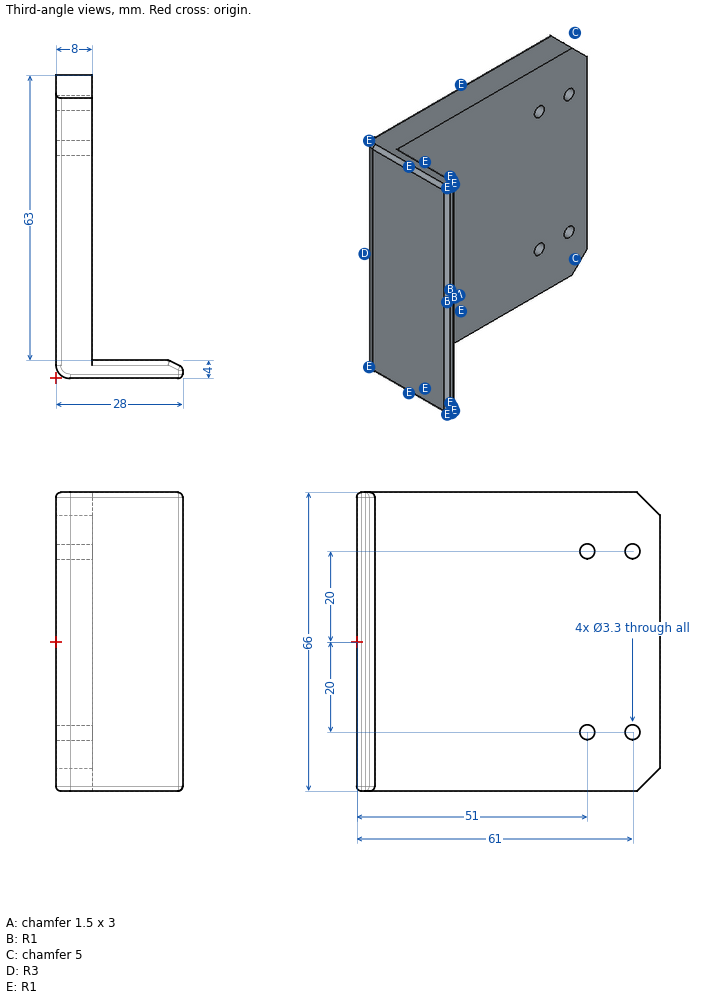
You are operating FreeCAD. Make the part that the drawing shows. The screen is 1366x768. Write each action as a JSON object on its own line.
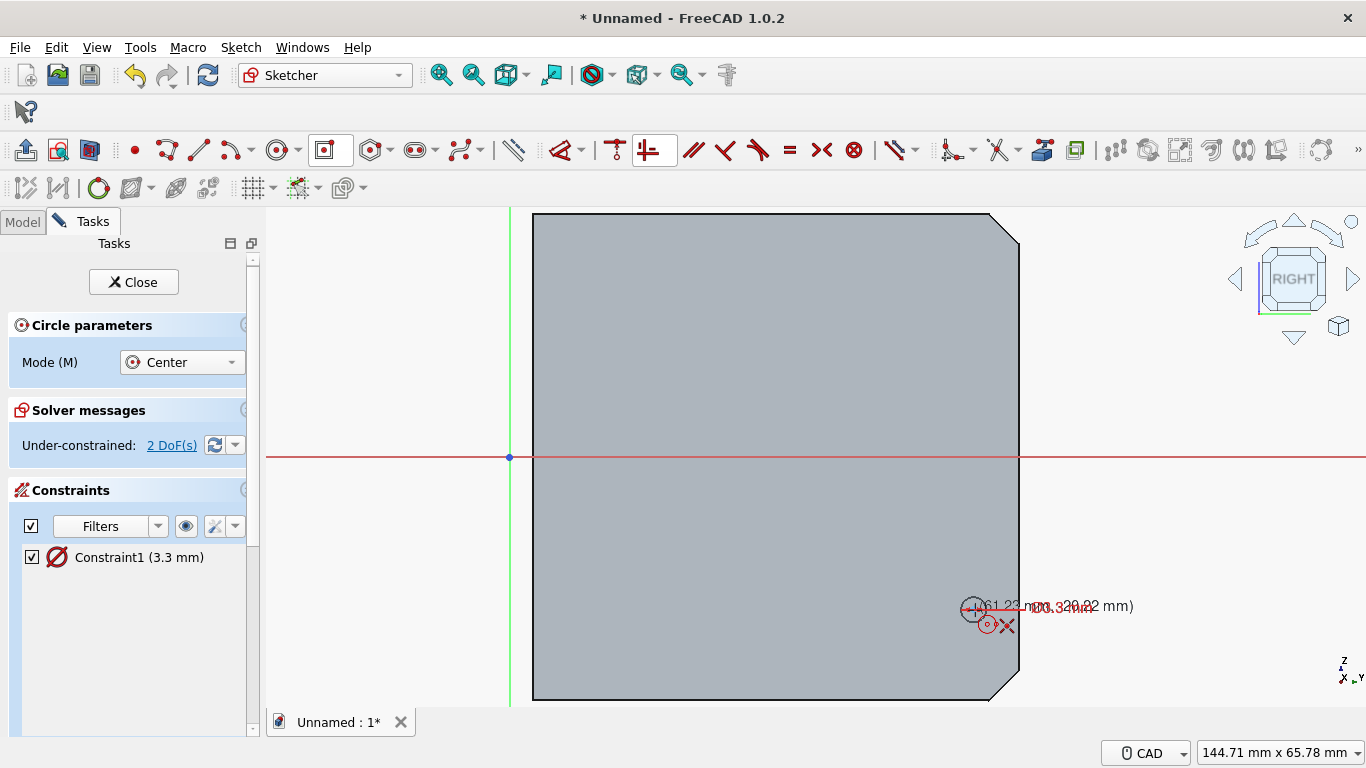
{"action": "scroll", "coordinate": [974, 305], "scroll_direction": "up", "scroll_amount": 3}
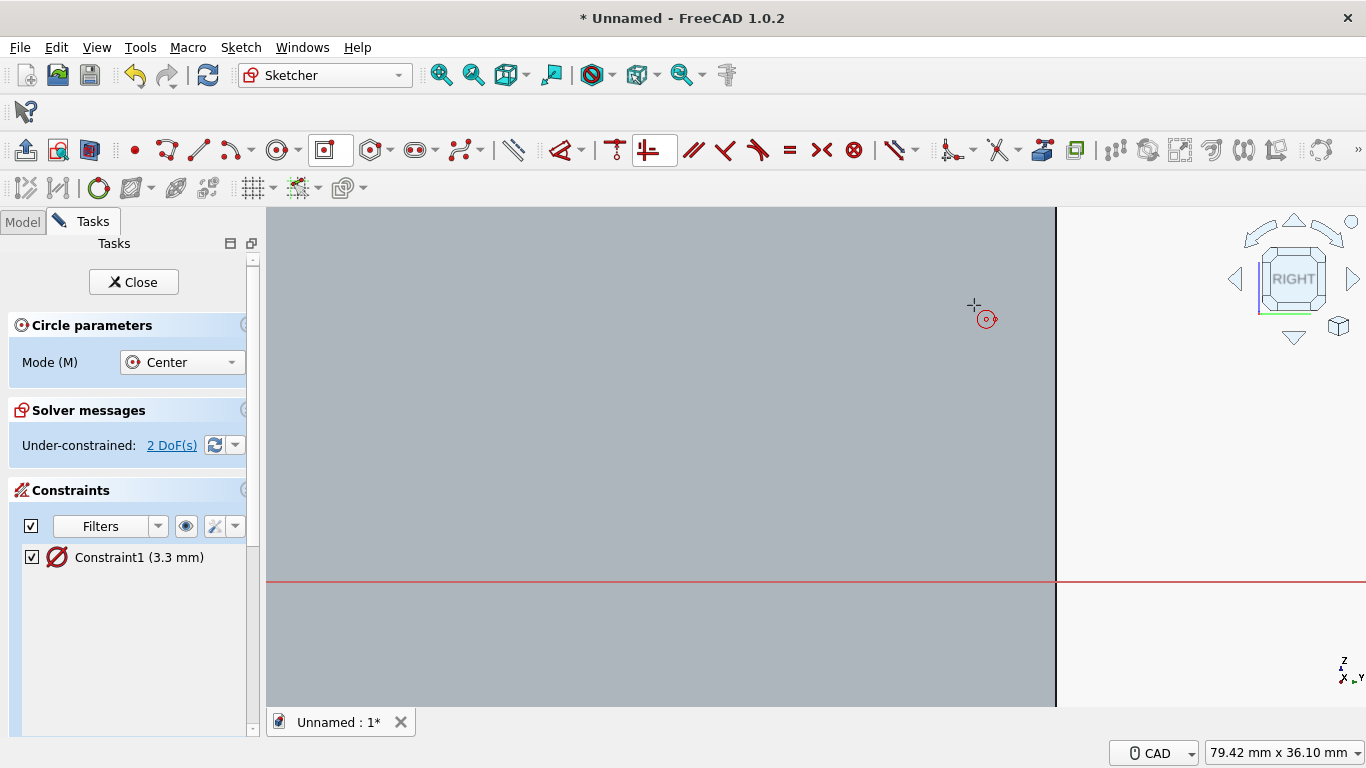
{"action": "left_click", "coordinate": [973, 305]}
{"action": "mouse_move", "coordinate": [989, 289]}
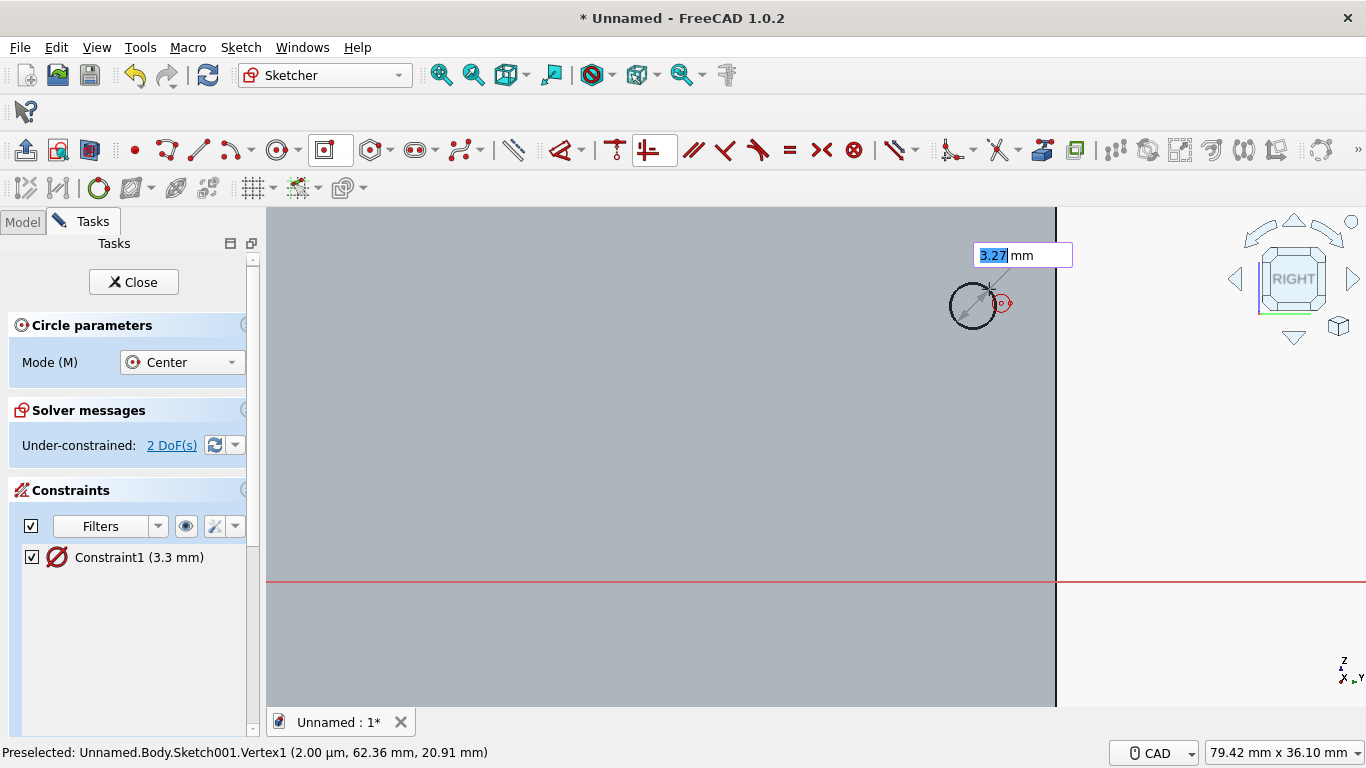
{"action": "type", "text": "3.3"}
{"action": "key", "text": "Return"}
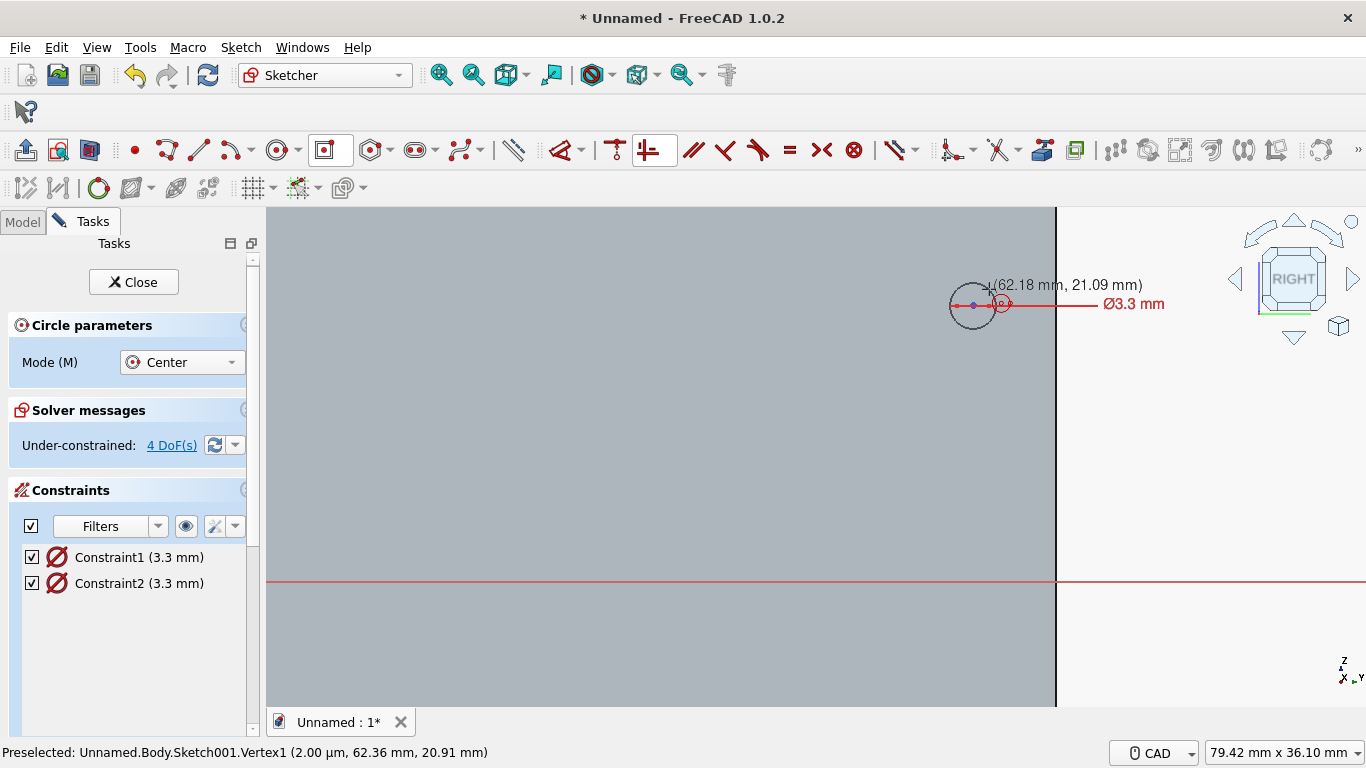
{"action": "scroll", "coordinate": [974, 305], "scroll_direction": "down", "scroll_amount": 3}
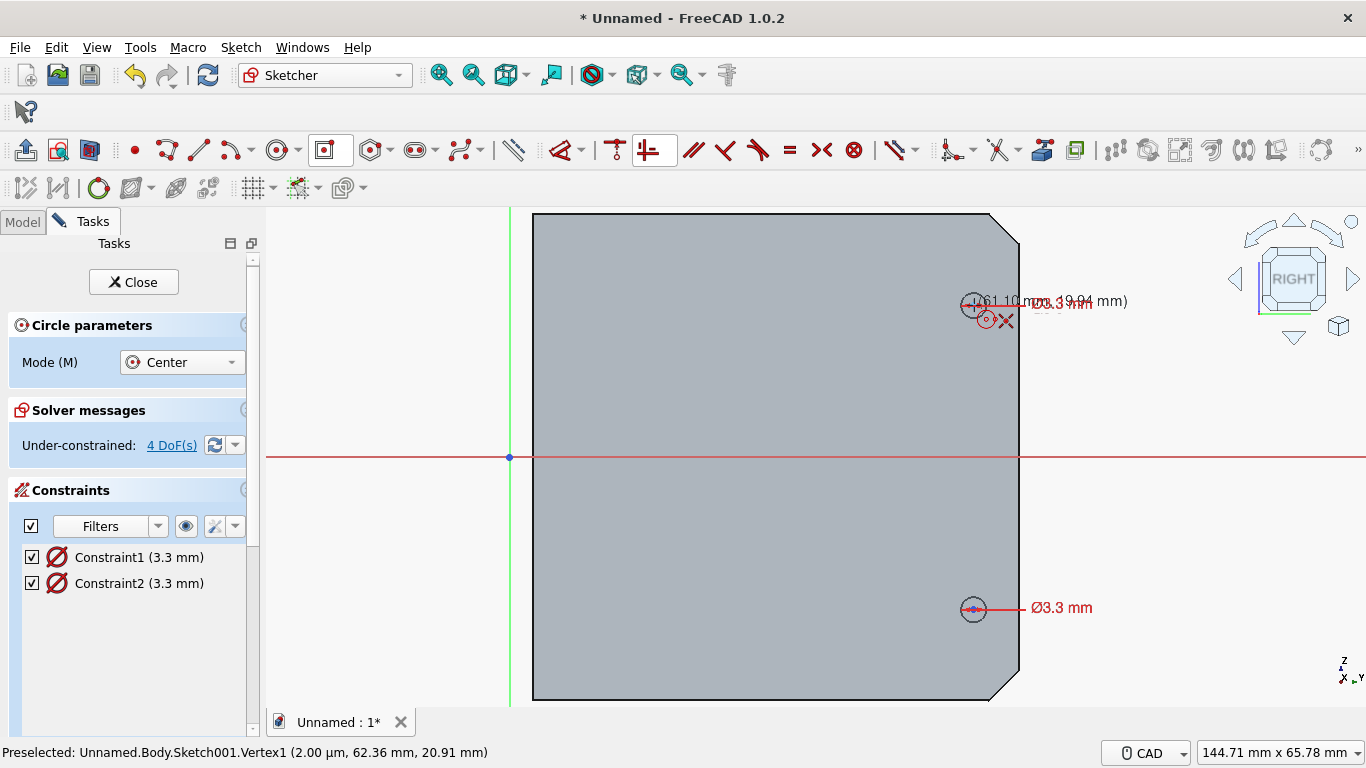
{"action": "scroll", "coordinate": [898, 609], "scroll_direction": "up", "scroll_amount": 3}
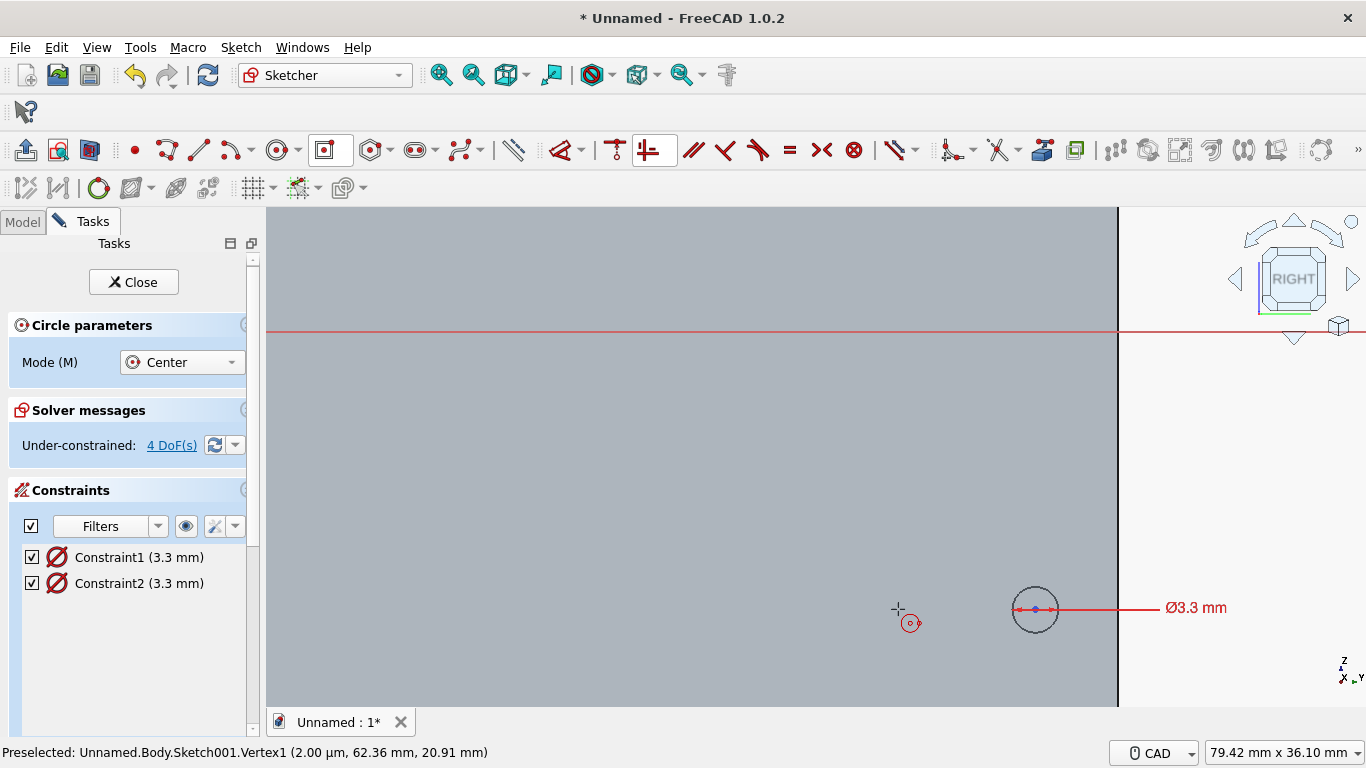
{"action": "left_click", "coordinate": [897, 609]}
{"action": "mouse_move", "coordinate": [913, 593]}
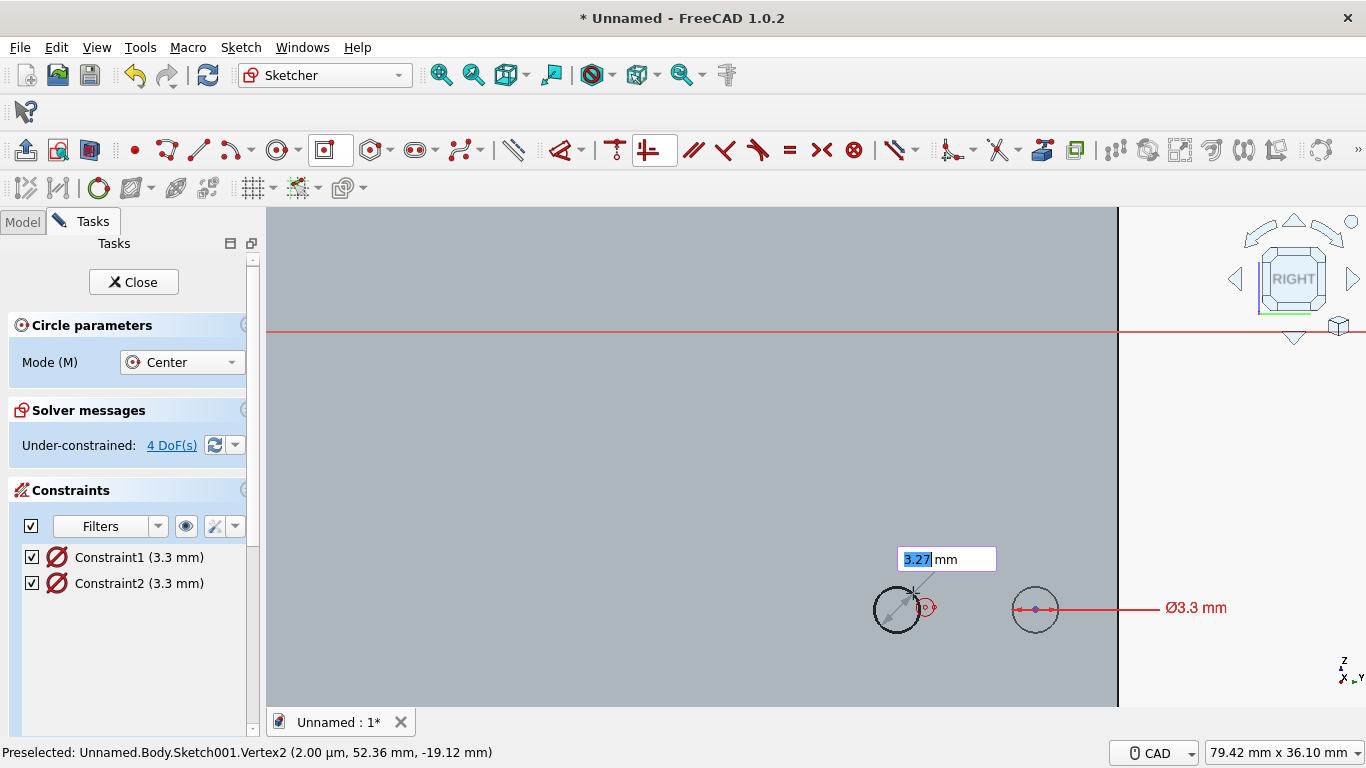
{"action": "type", "text": "3.3"}
{"action": "key", "text": "Return"}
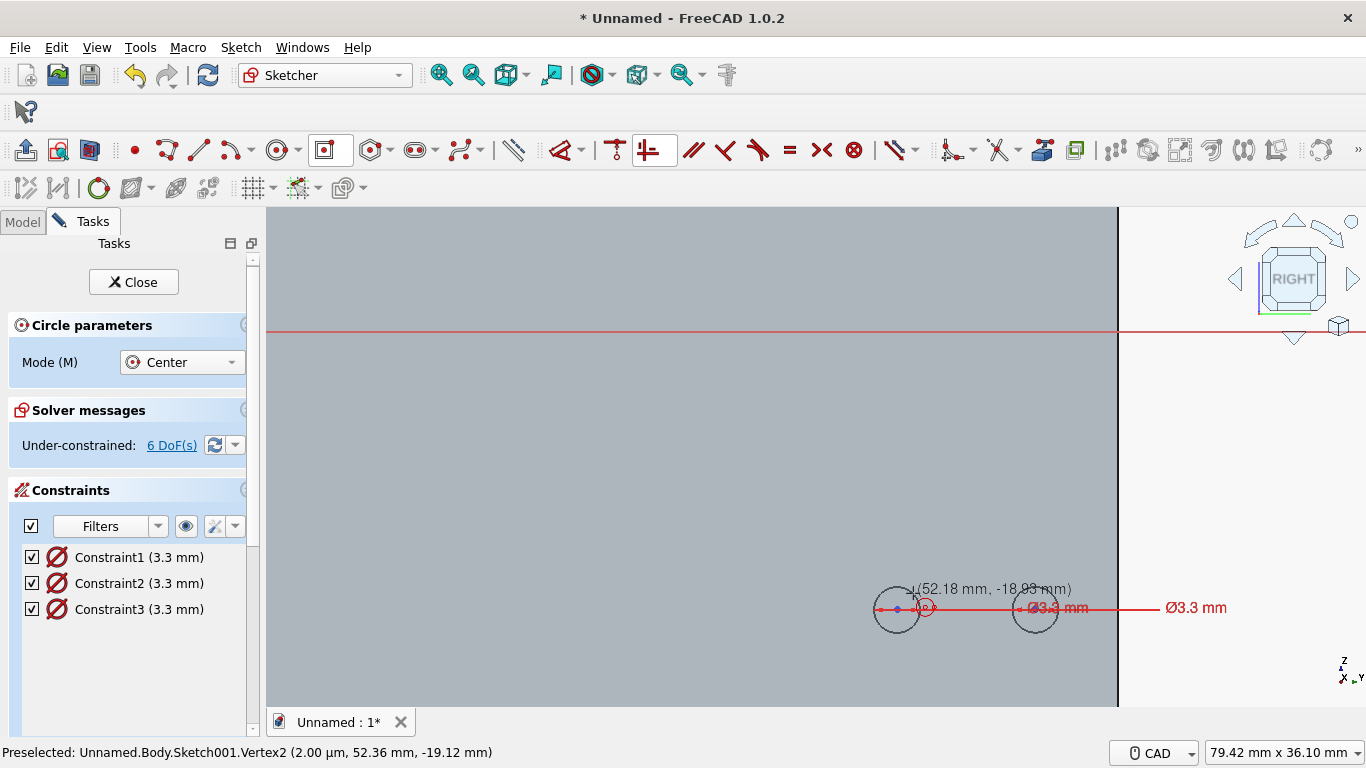
{"action": "scroll", "coordinate": [898, 609], "scroll_direction": "down", "scroll_amount": 3}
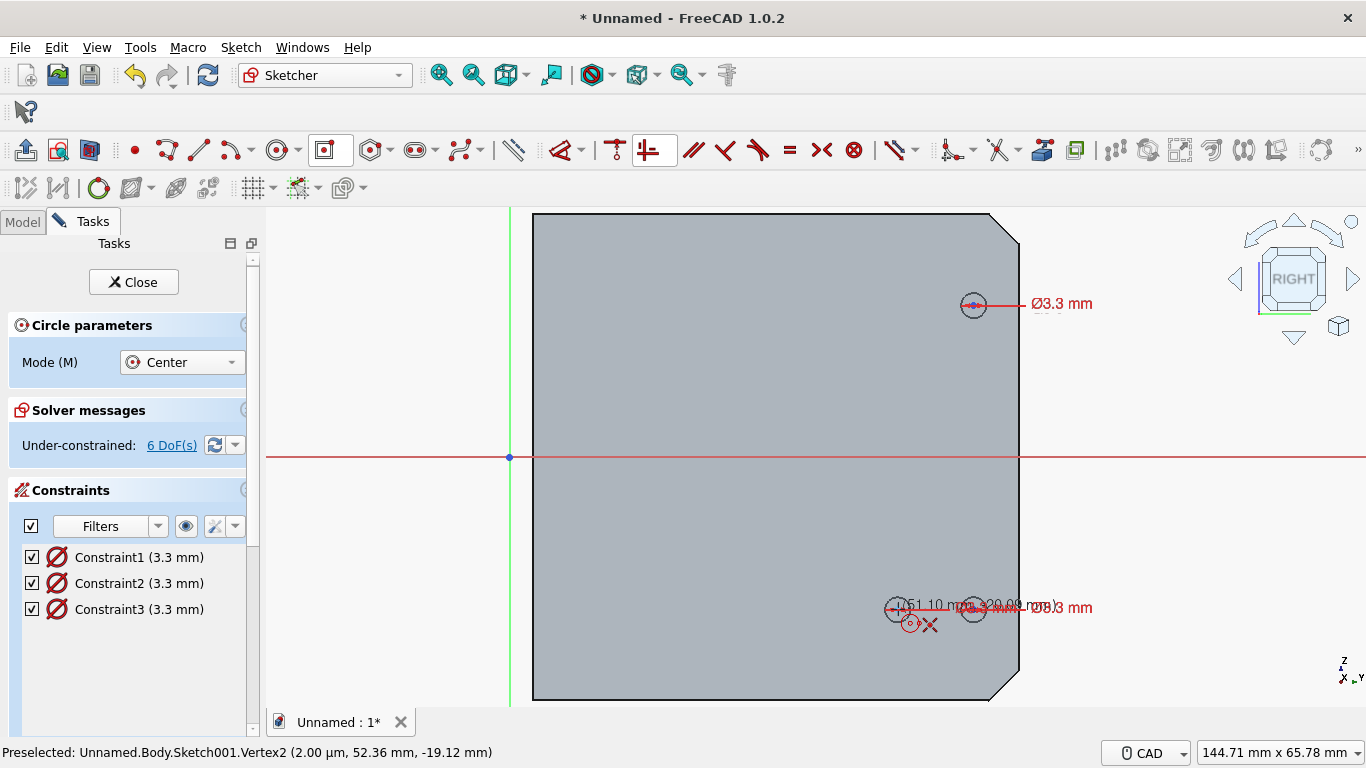
{"action": "scroll", "coordinate": [898, 305], "scroll_direction": "up", "scroll_amount": 3}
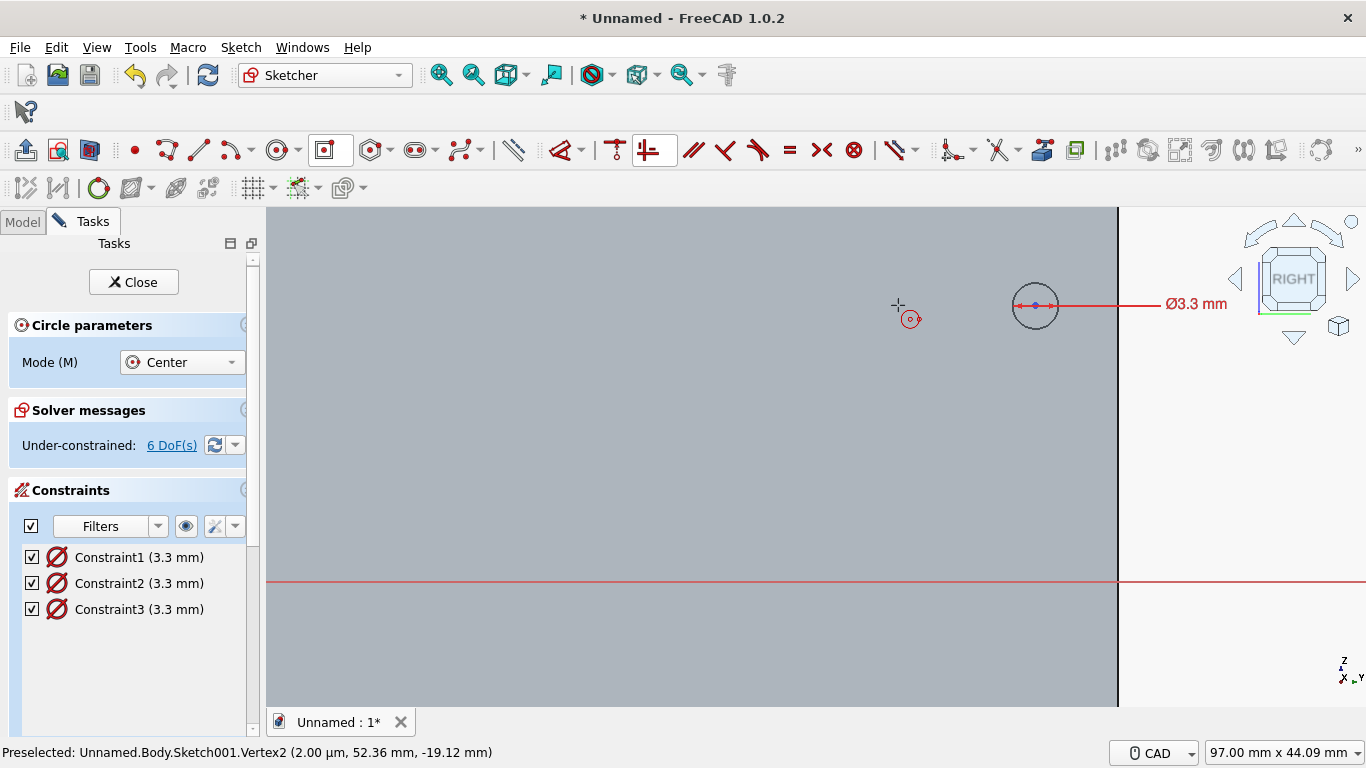
{"action": "left_click", "coordinate": [897, 305]}
{"action": "mouse_move", "coordinate": [913, 289]}